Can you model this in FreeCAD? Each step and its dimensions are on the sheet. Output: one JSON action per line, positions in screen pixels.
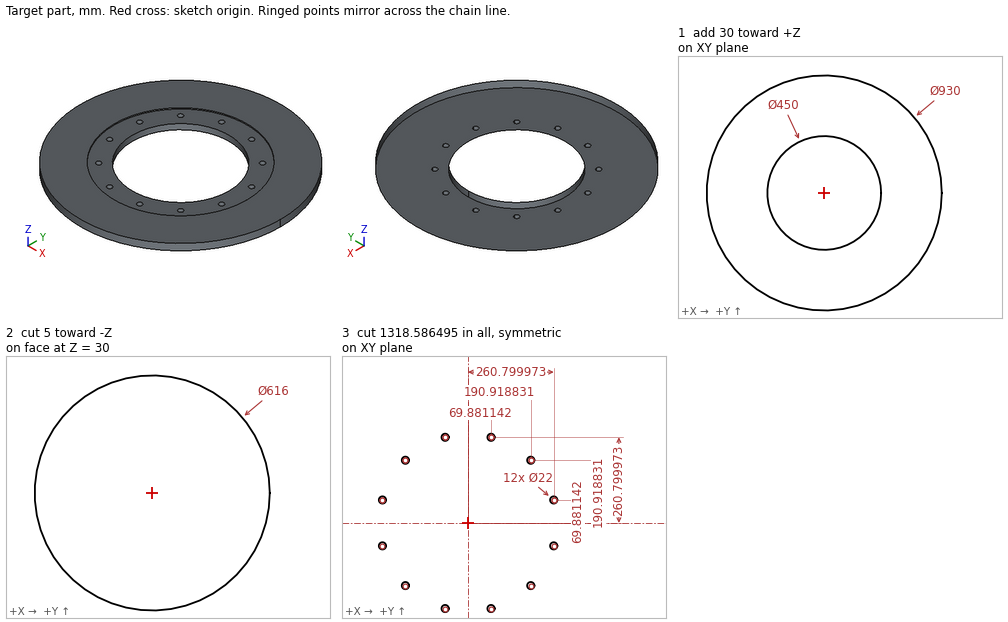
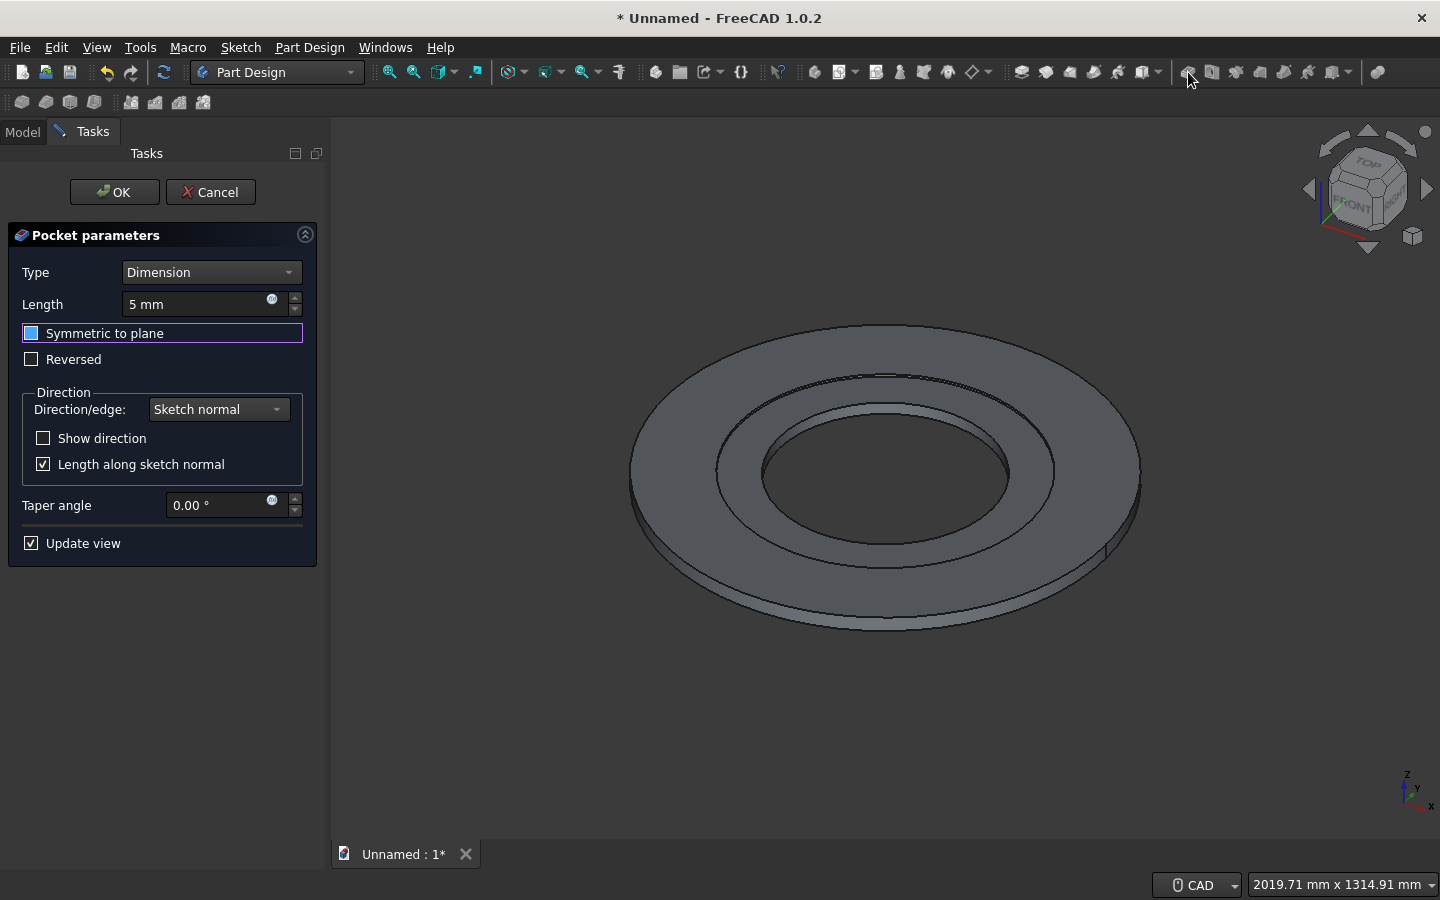
{"action": "left_click", "coordinate": [115, 192]}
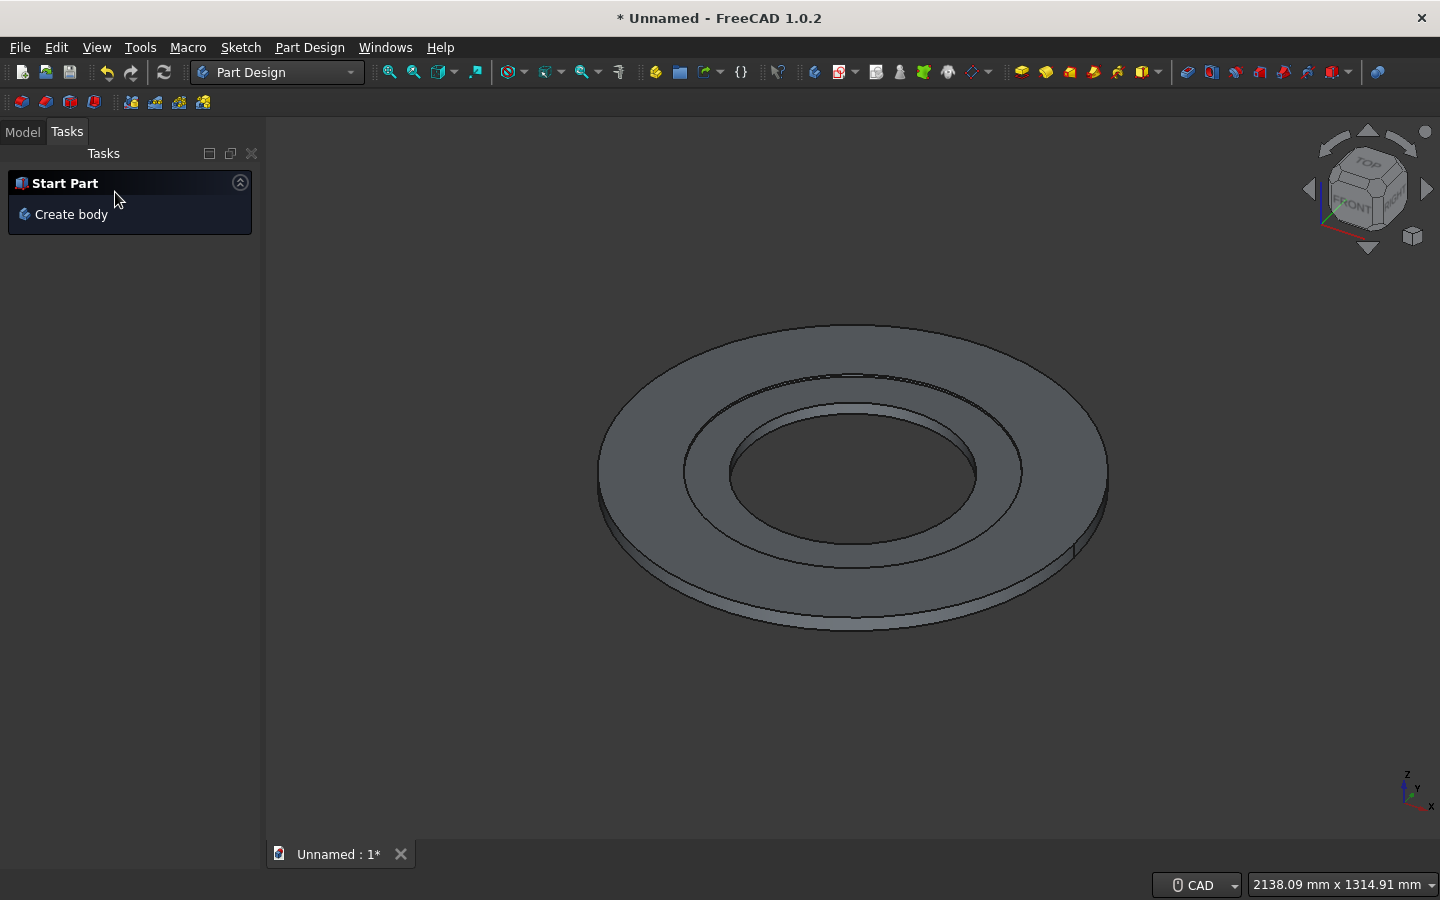
{"action": "left_click", "coordinate": [840, 72]}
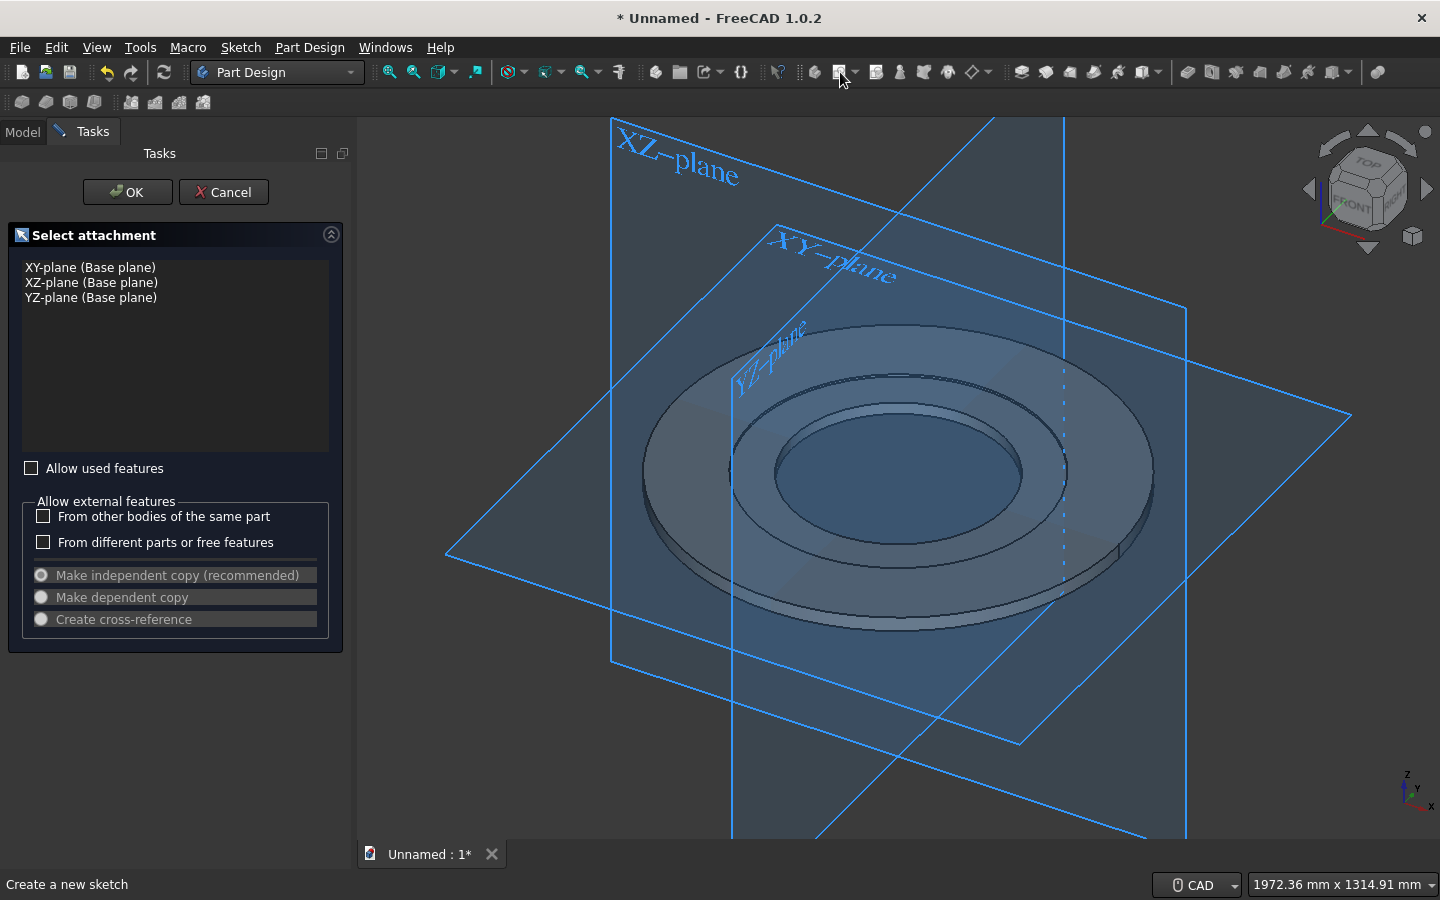
{"action": "left_click", "coordinate": [82, 268]}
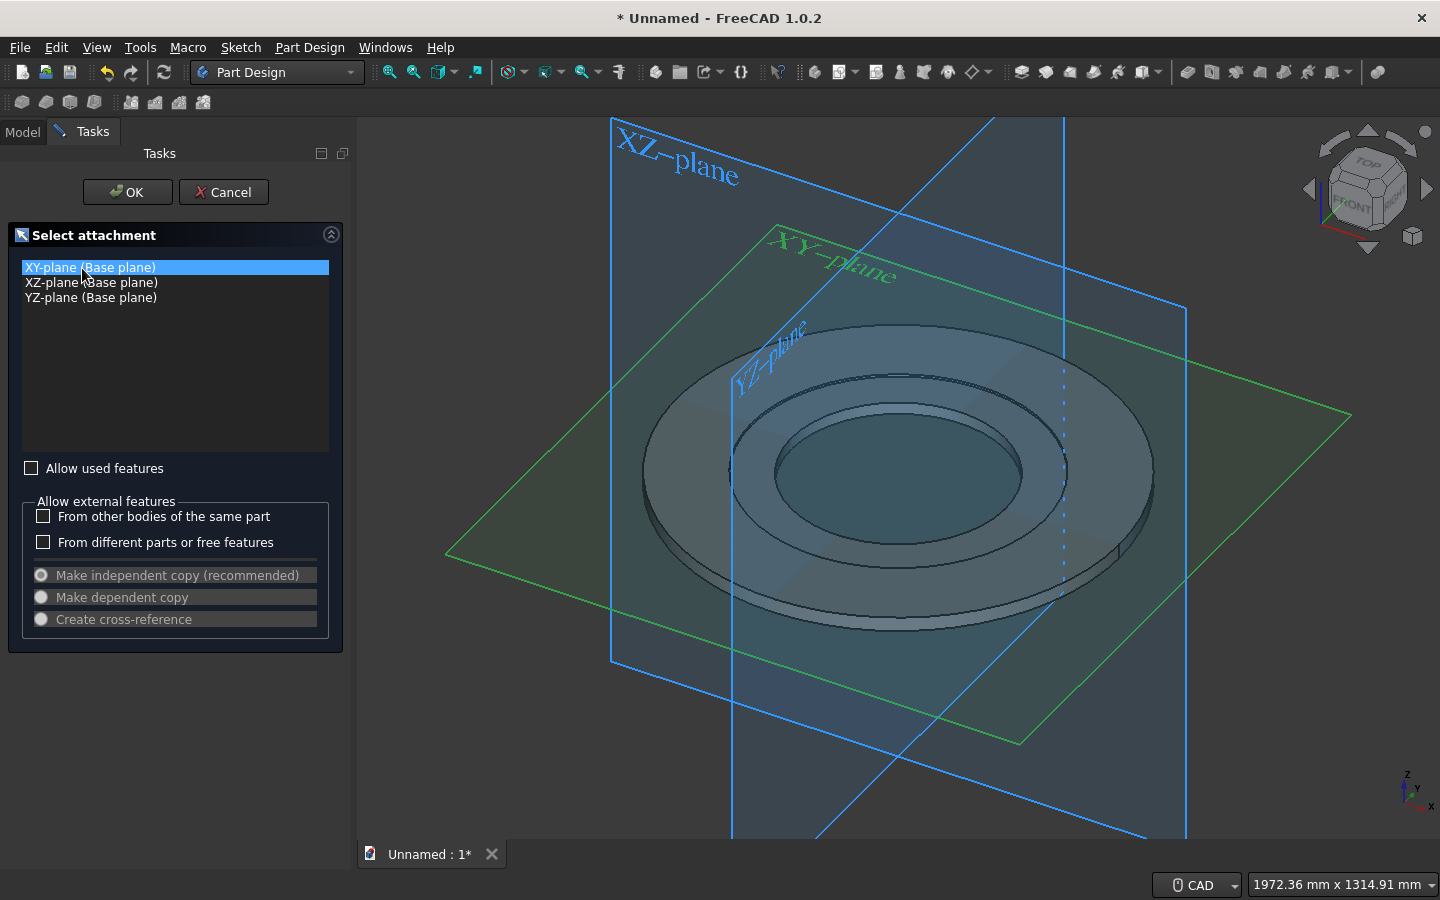
{"action": "left_click", "coordinate": [128, 192]}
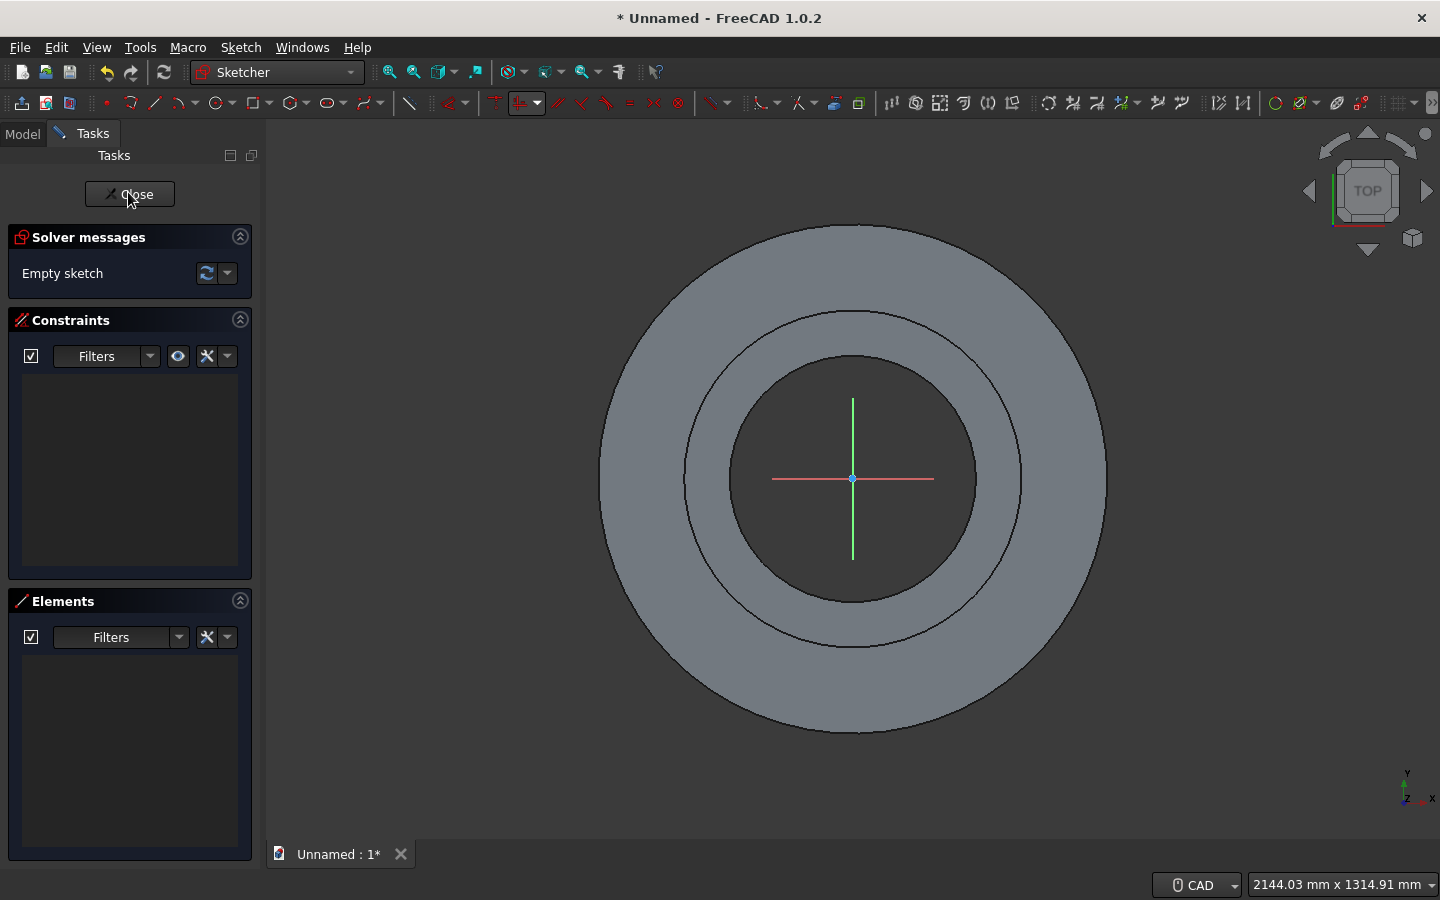
{"action": "left_click", "coordinate": [70, 104]}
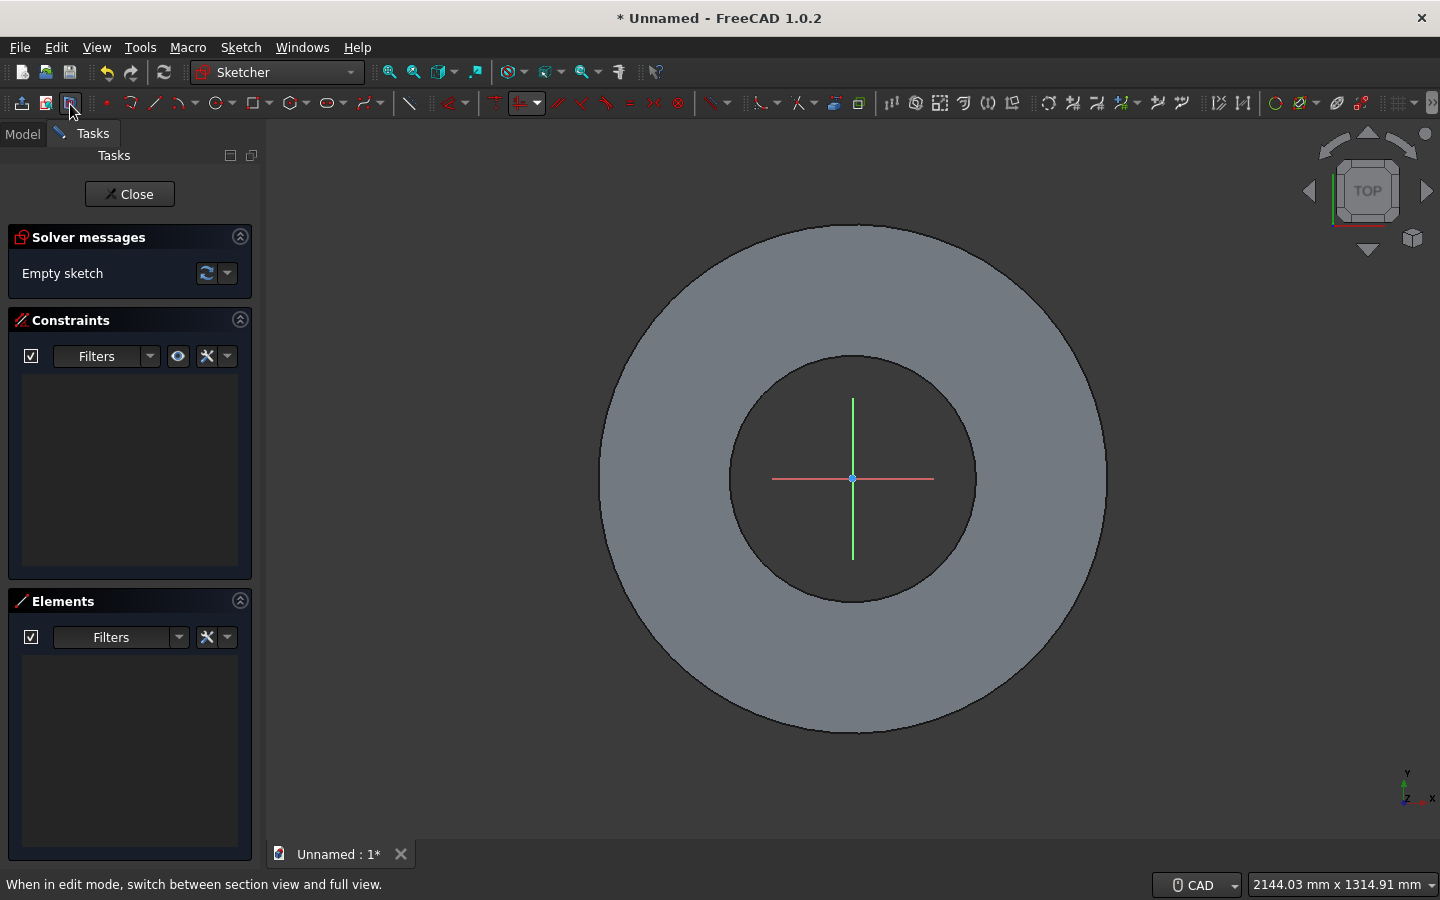
{"action": "scroll", "coordinate": [992, 479], "scroll_direction": "up", "scroll_amount": 2}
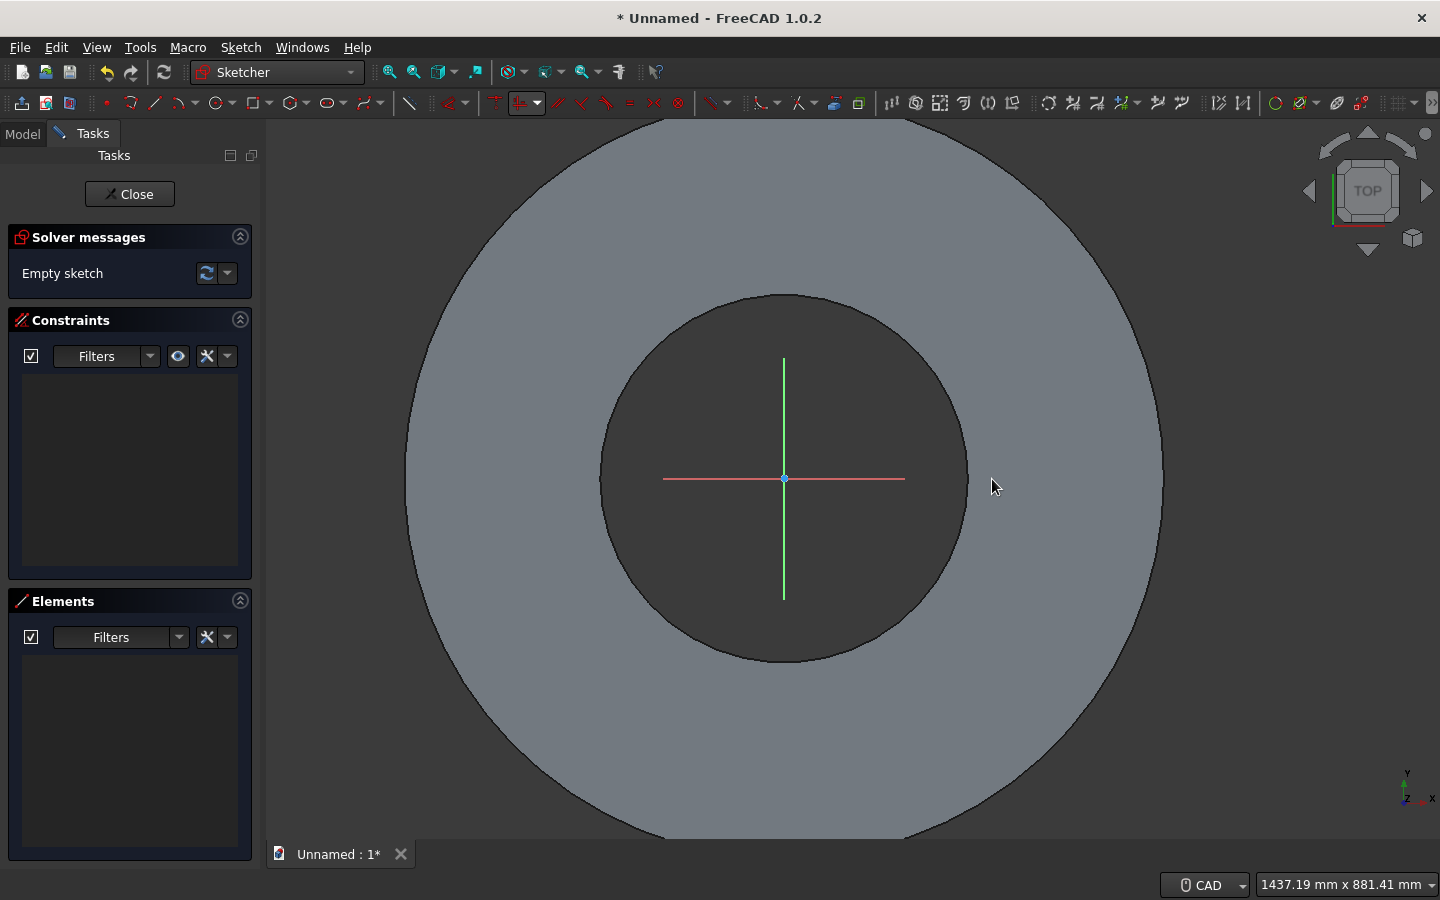
{"action": "left_click", "coordinate": [216, 104]}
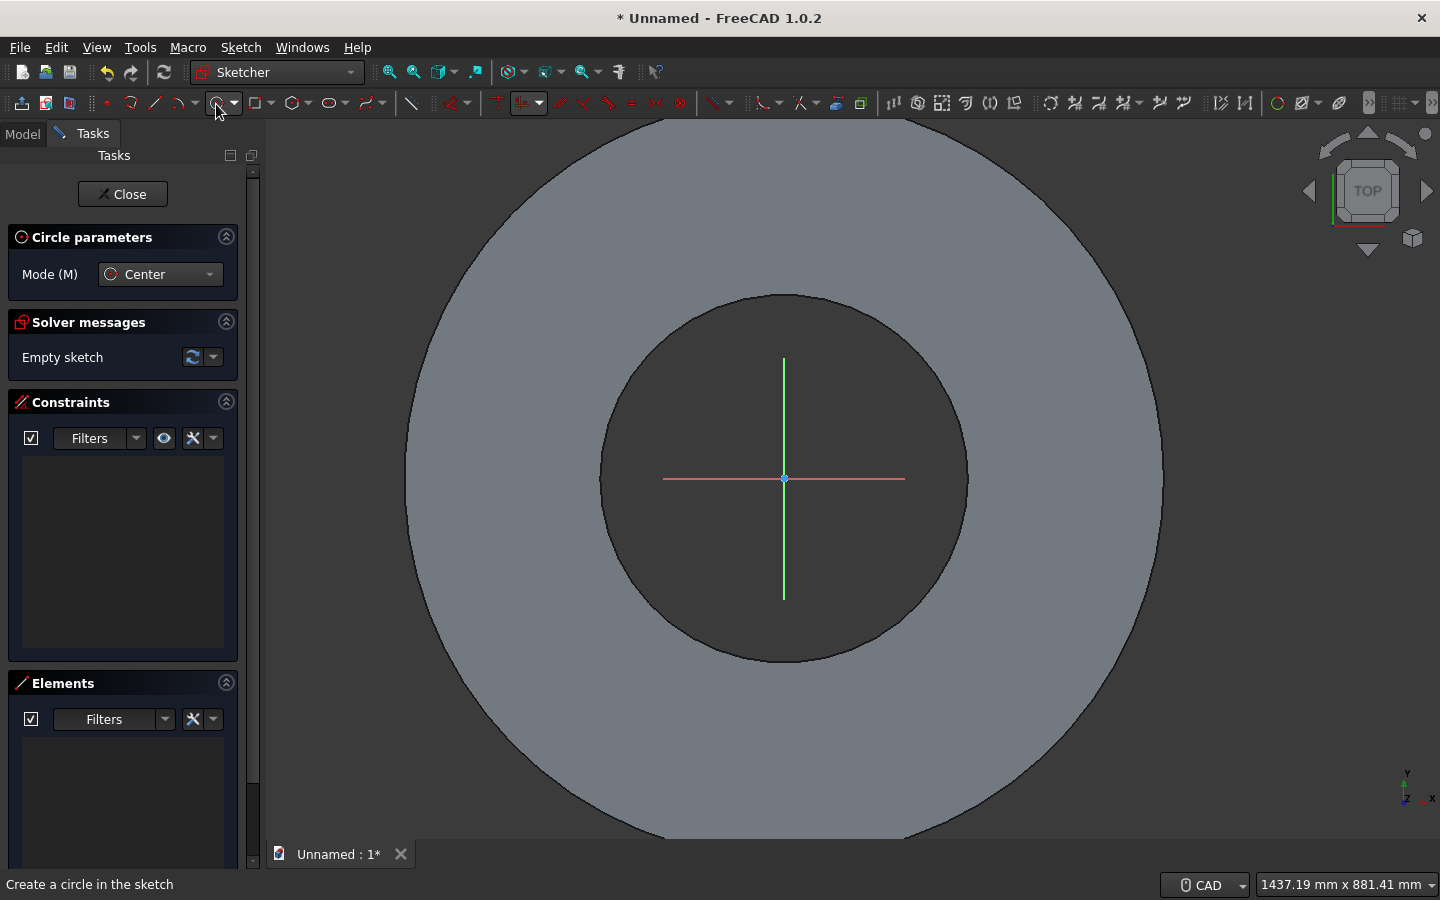
{"action": "scroll", "coordinate": [997, 422], "scroll_direction": "up", "scroll_amount": 5}